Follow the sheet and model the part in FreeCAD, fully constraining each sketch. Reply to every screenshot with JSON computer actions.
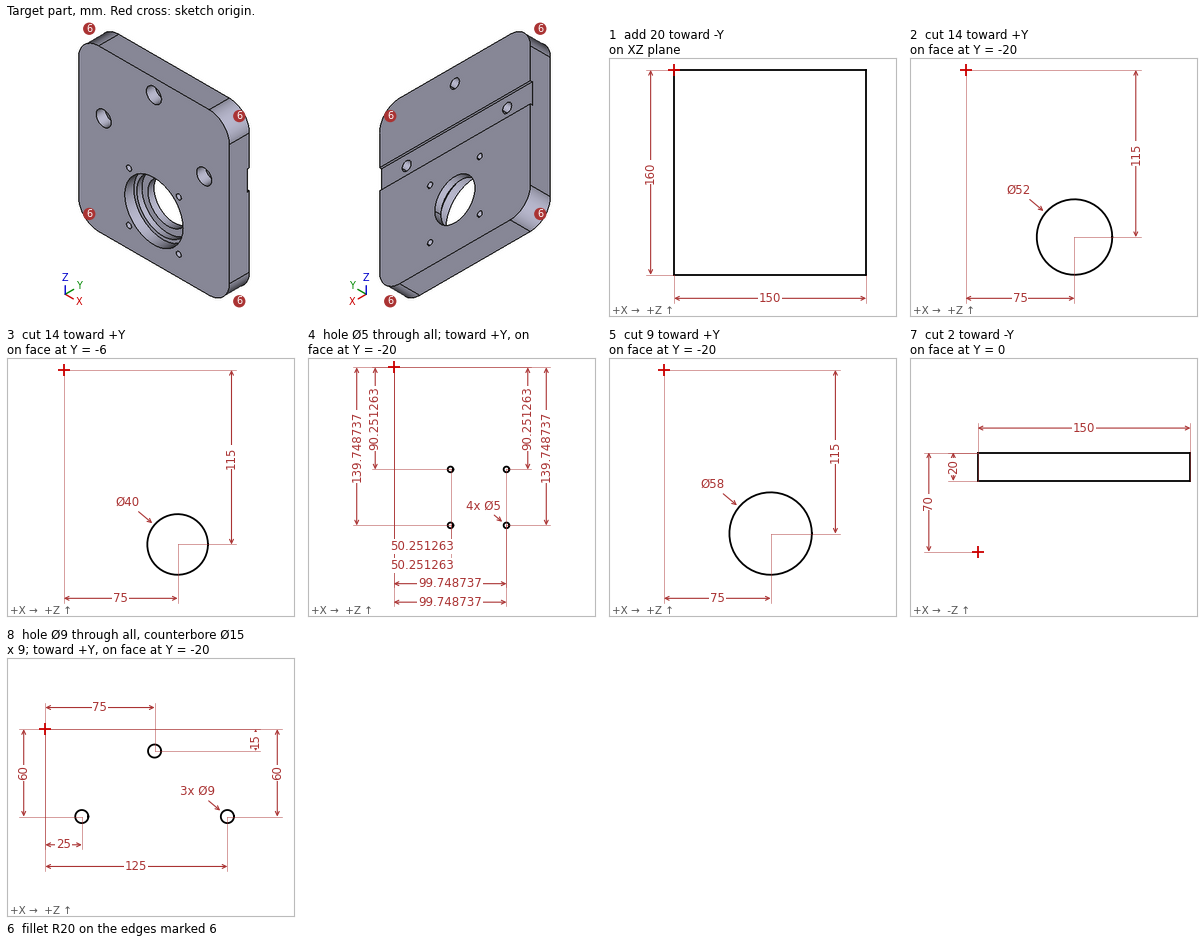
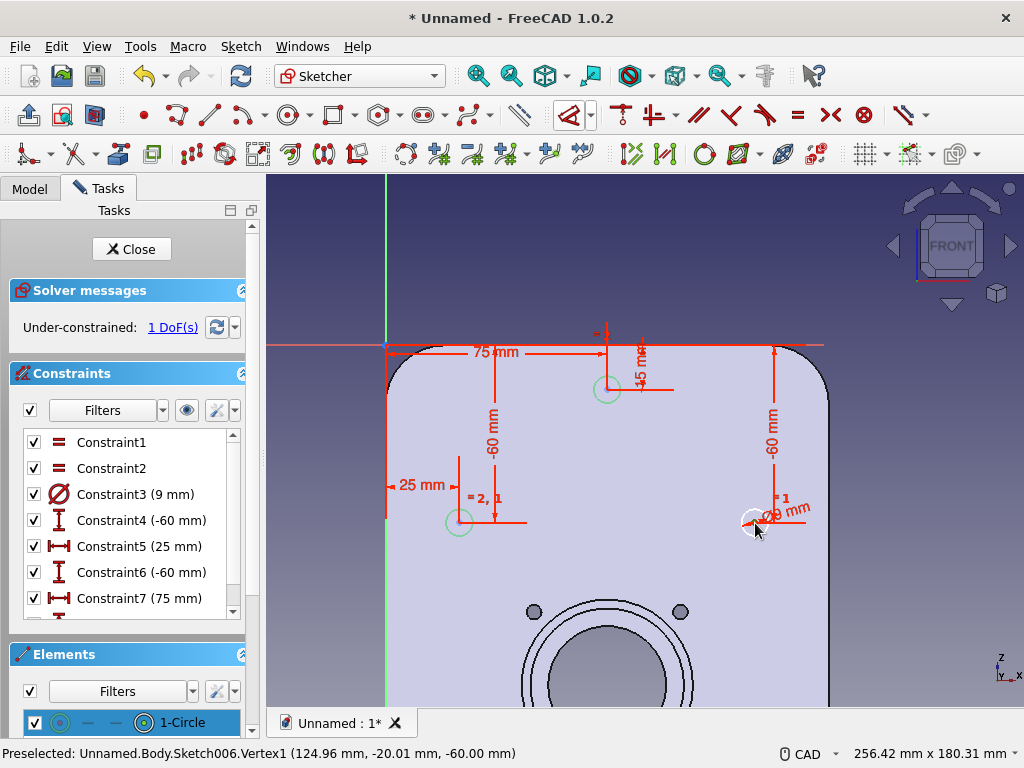
{"action": "left_click", "coordinate": [590, 116]}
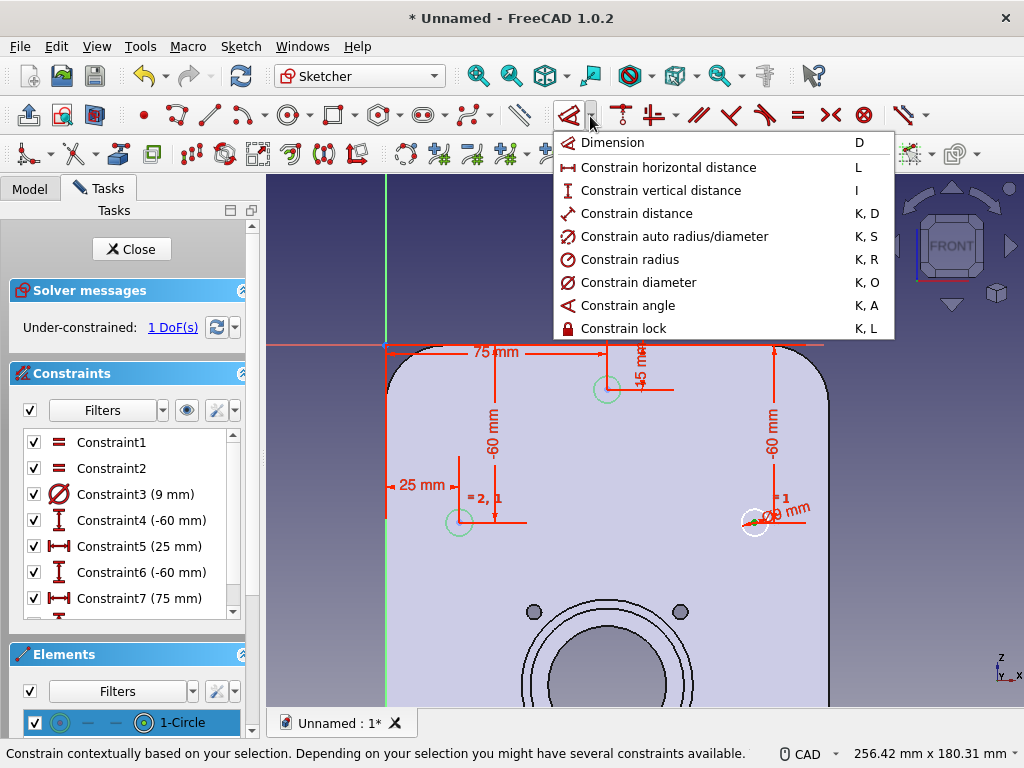
{"action": "left_click", "coordinate": [724, 168]}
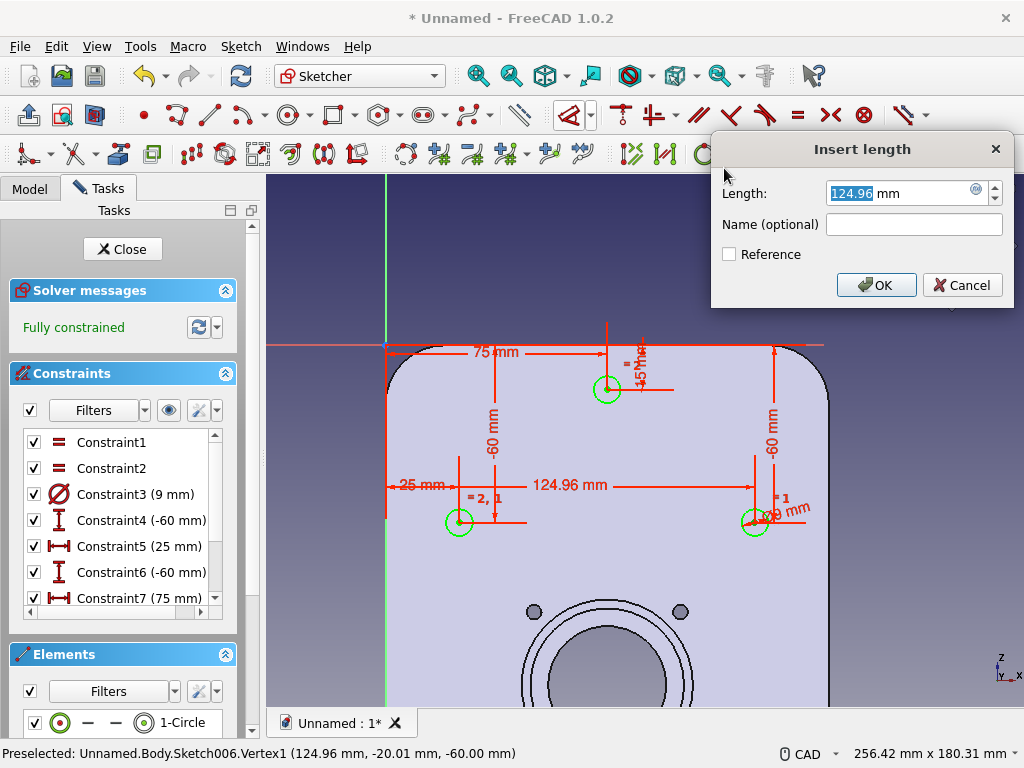
{"action": "type", "text": "125"}
{"action": "key", "text": "Return"}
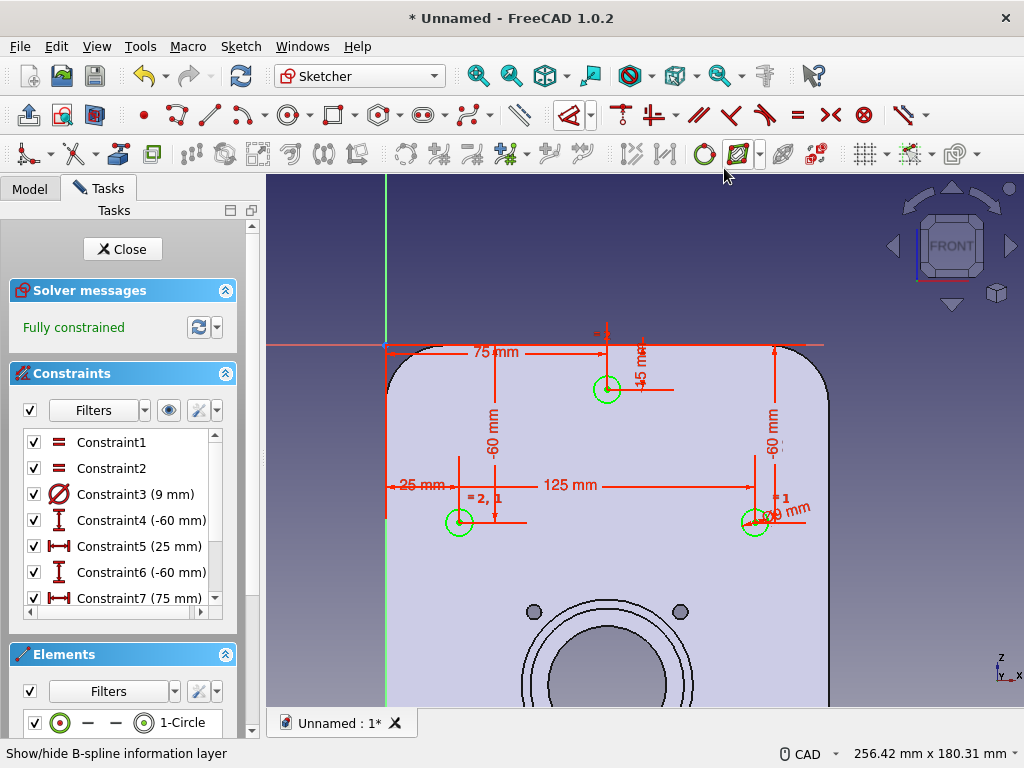
{"action": "left_click", "coordinate": [123, 249]}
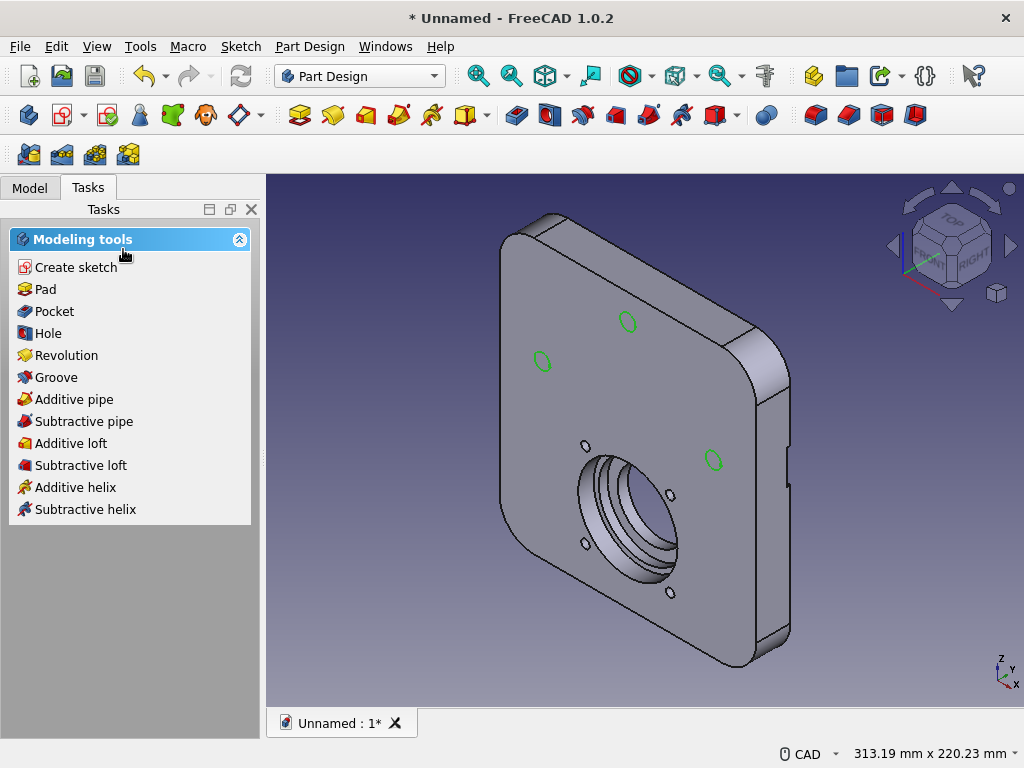
{"action": "left_click", "coordinate": [550, 116]}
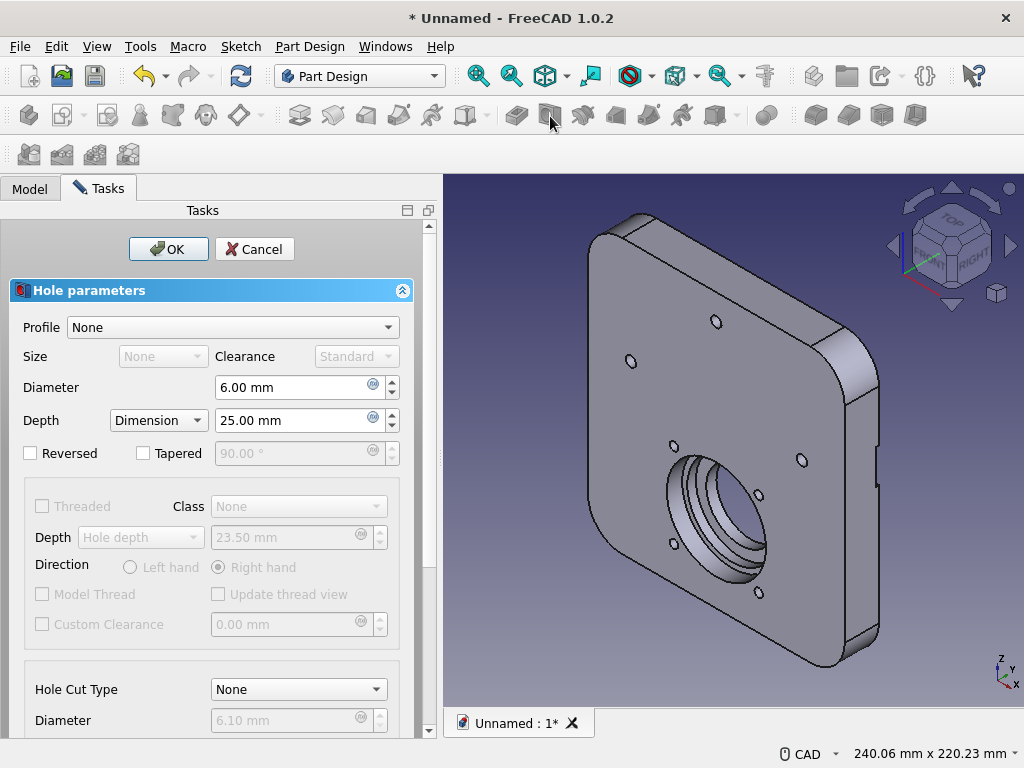
{"action": "triple_click", "coordinate": [300, 388]}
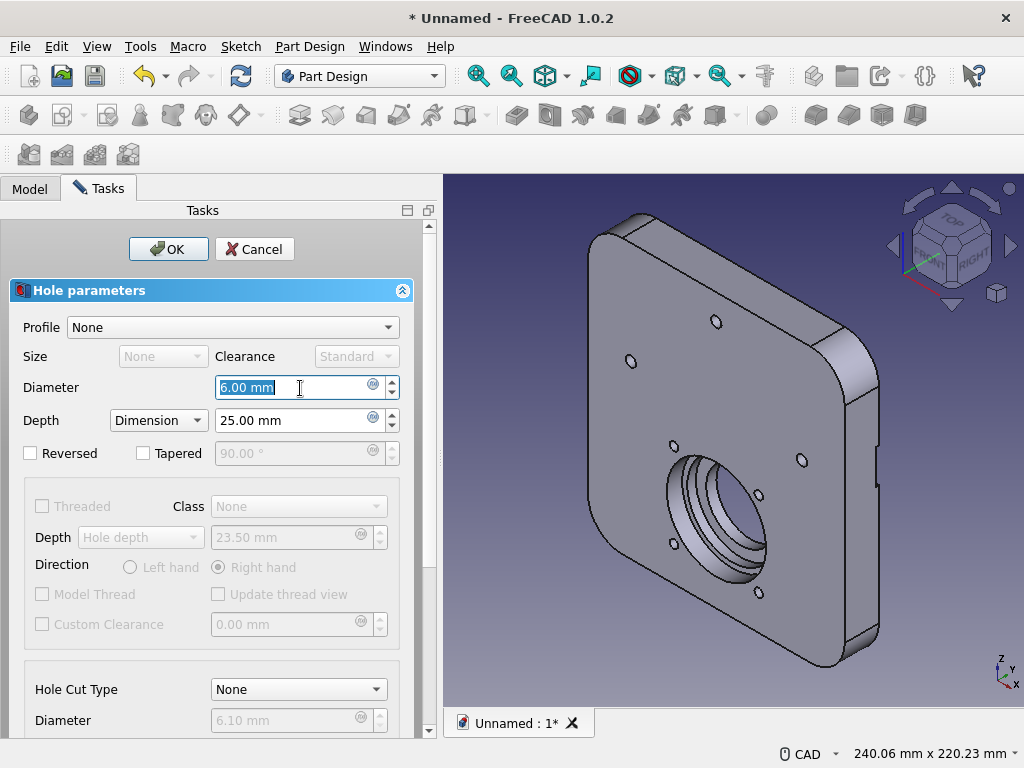
{"action": "type", "text": "9"}
{"action": "key", "text": "Tab"}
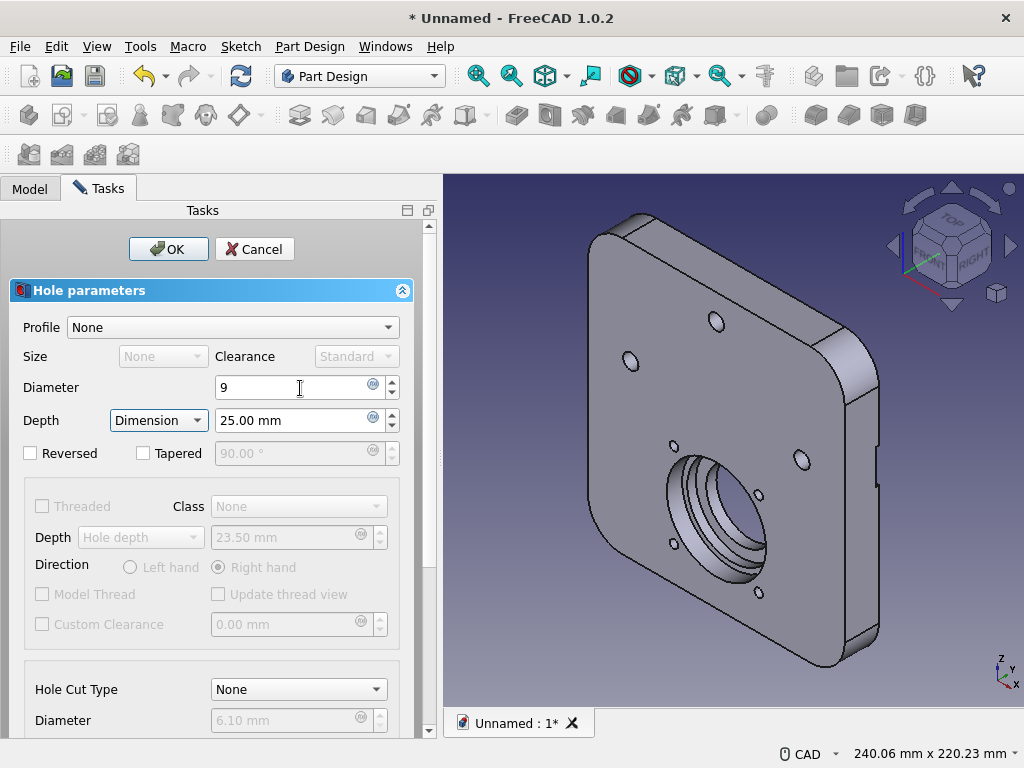
{"action": "left_click", "coordinate": [160, 420]}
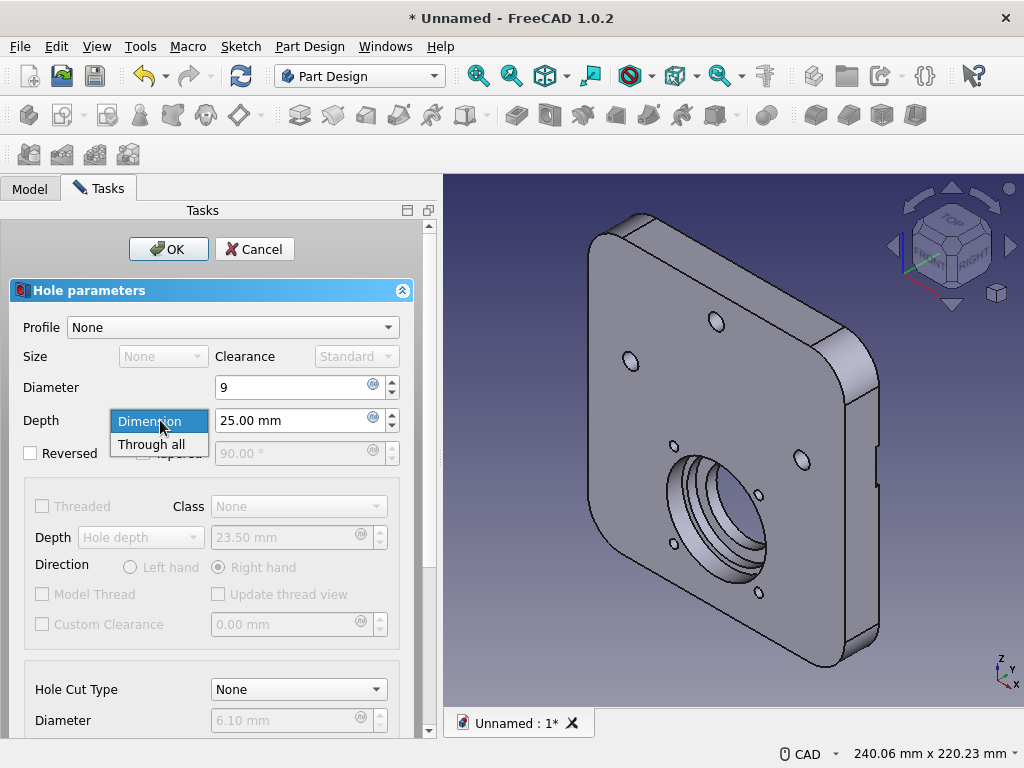
{"action": "left_click", "coordinate": [158, 444]}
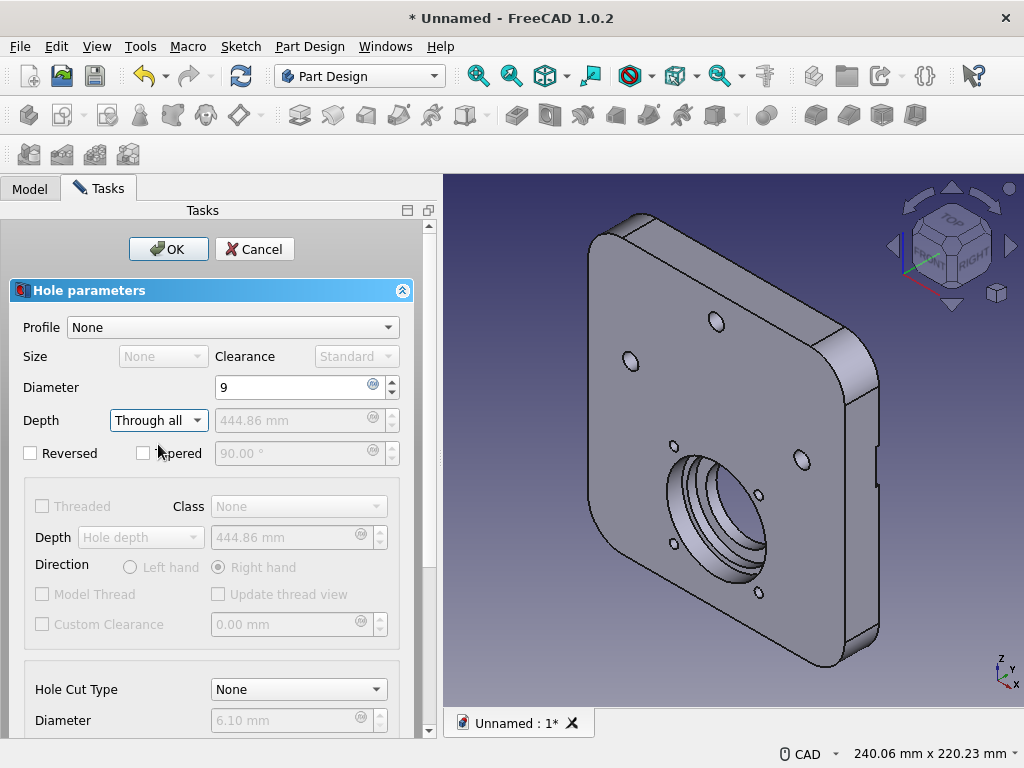
{"action": "left_click", "coordinate": [300, 690]}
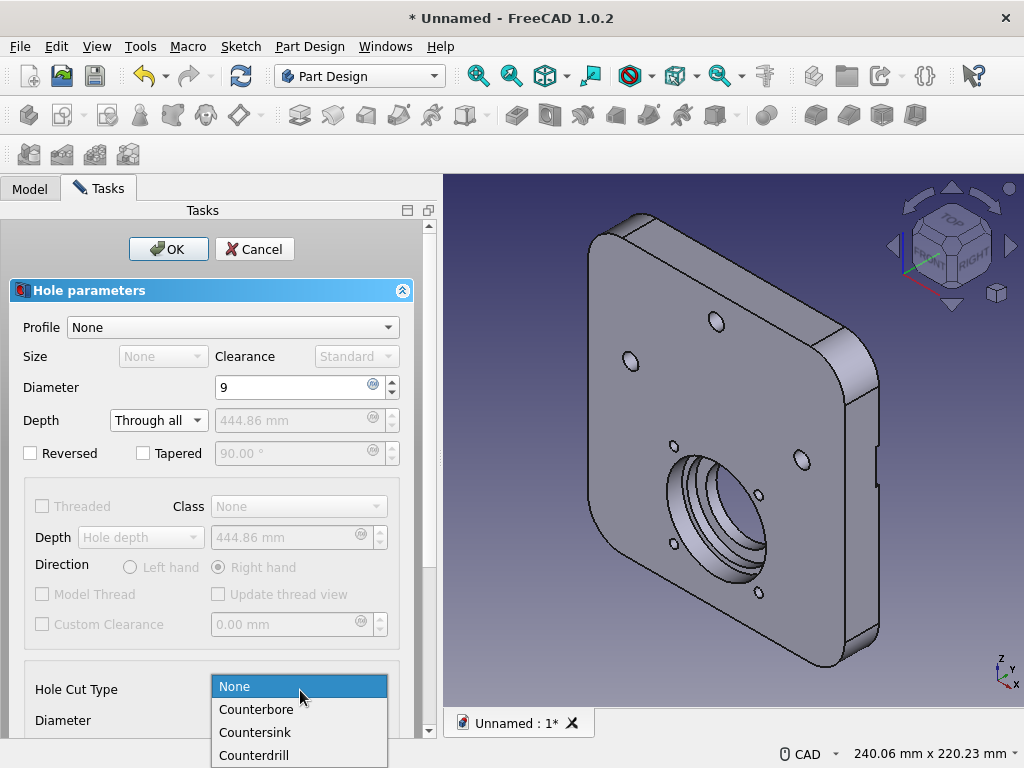
{"action": "left_click", "coordinate": [298, 710]}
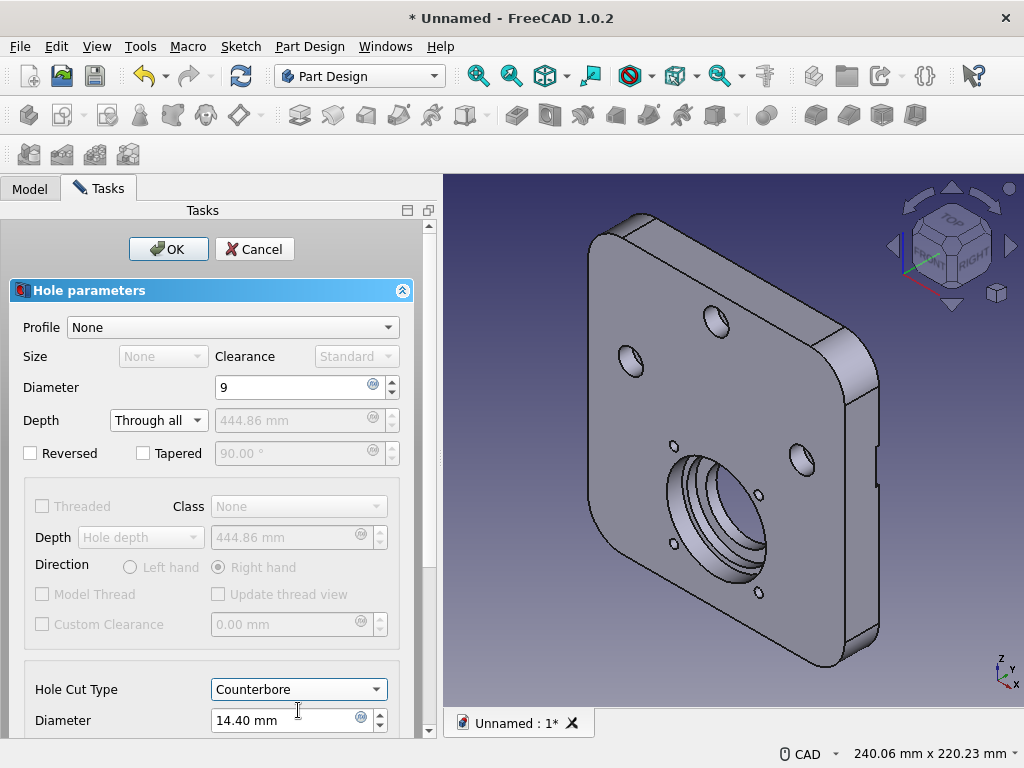
{"action": "triple_click", "coordinate": [292, 720]}